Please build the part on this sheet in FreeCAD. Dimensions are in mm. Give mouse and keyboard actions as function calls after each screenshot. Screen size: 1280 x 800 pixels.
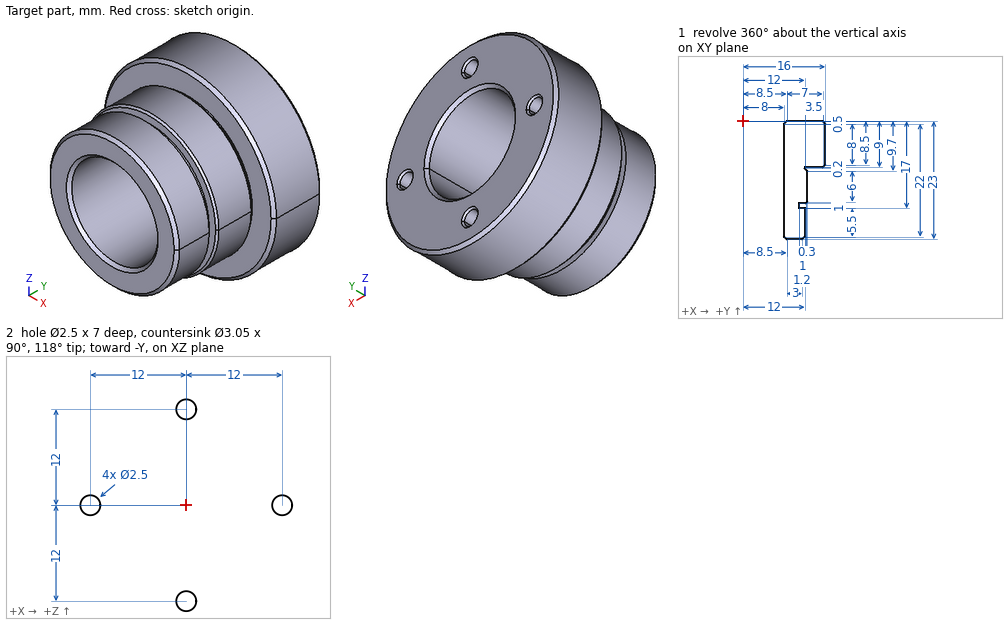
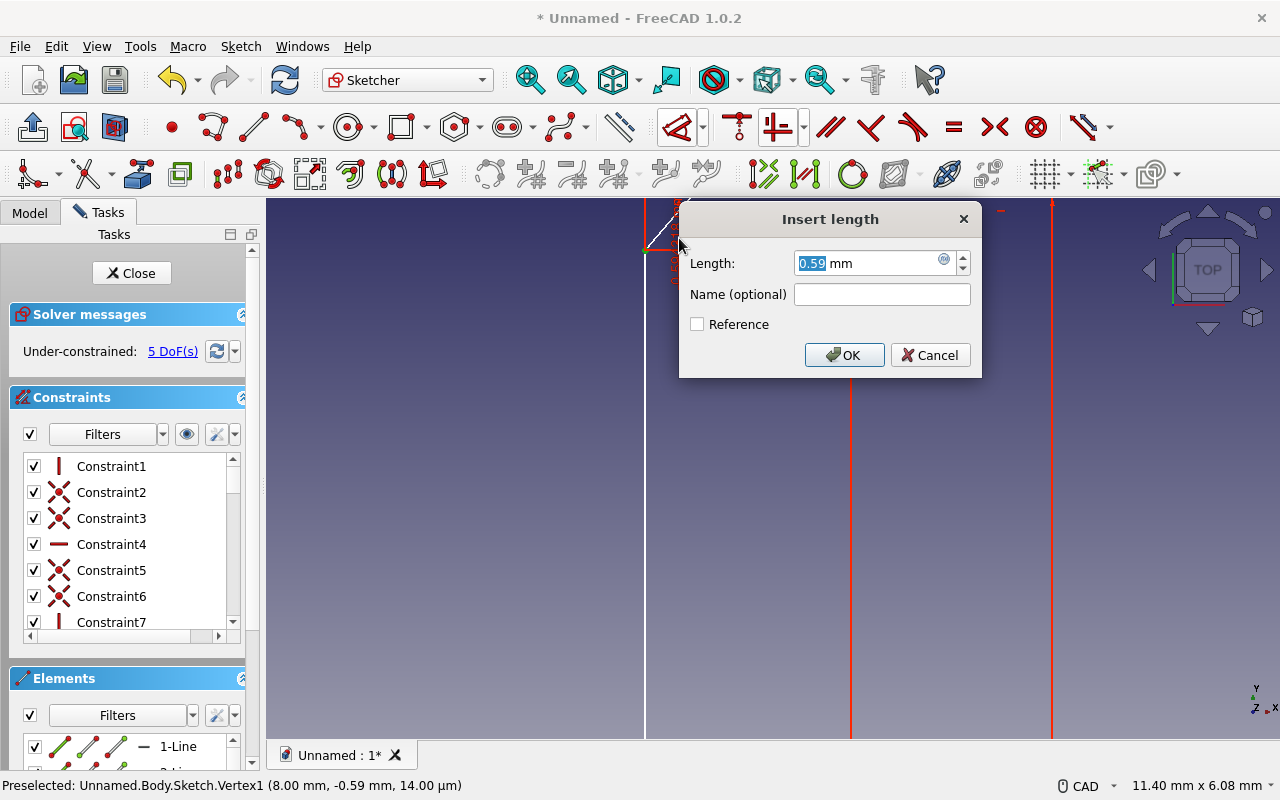
text(0.5)
key(Return)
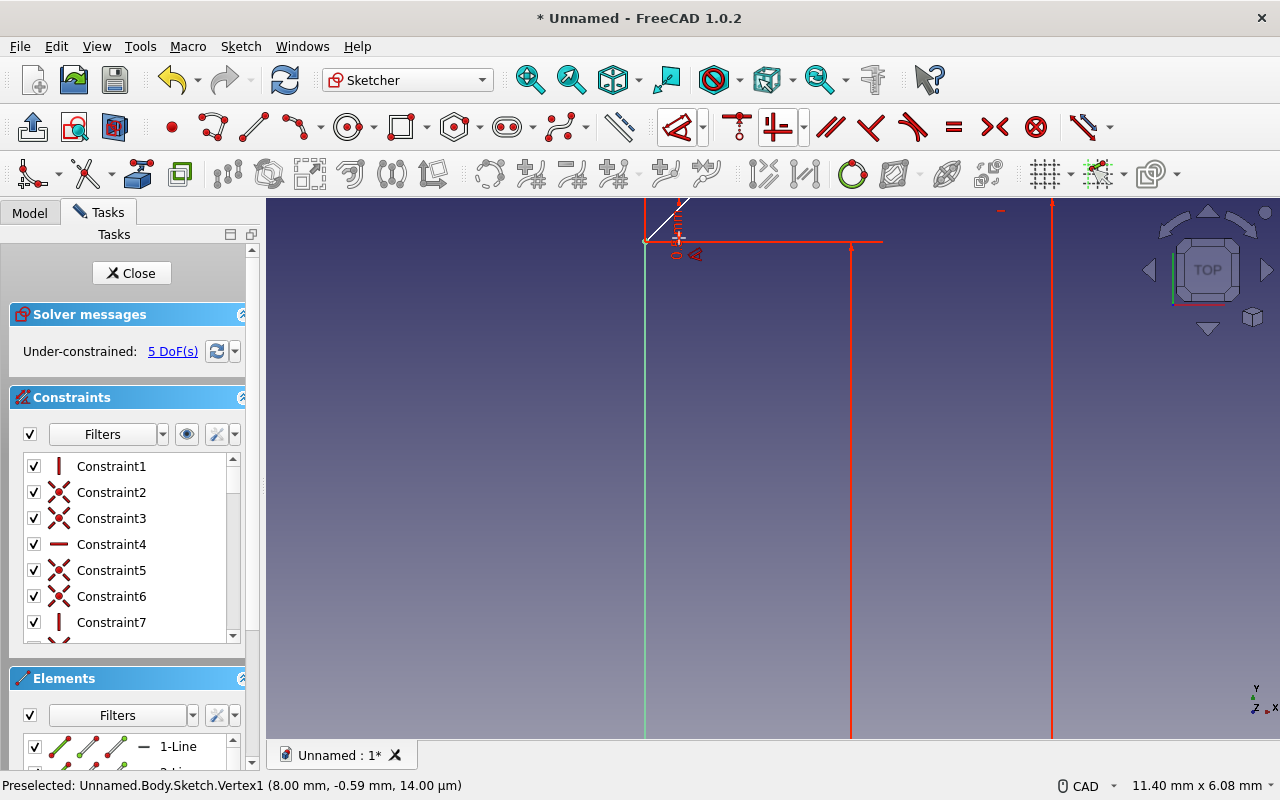
scroll(716, 320, down, 9)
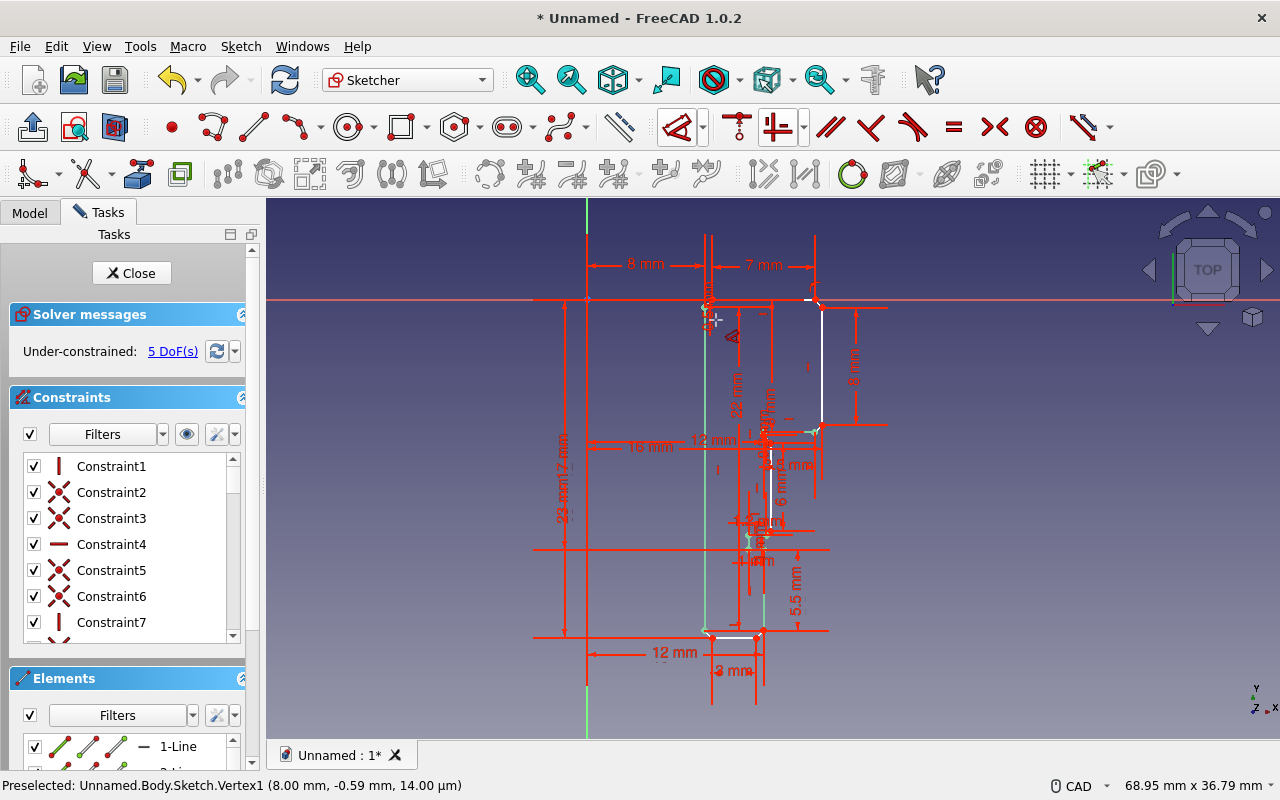
click(712, 638)
click(650, 696)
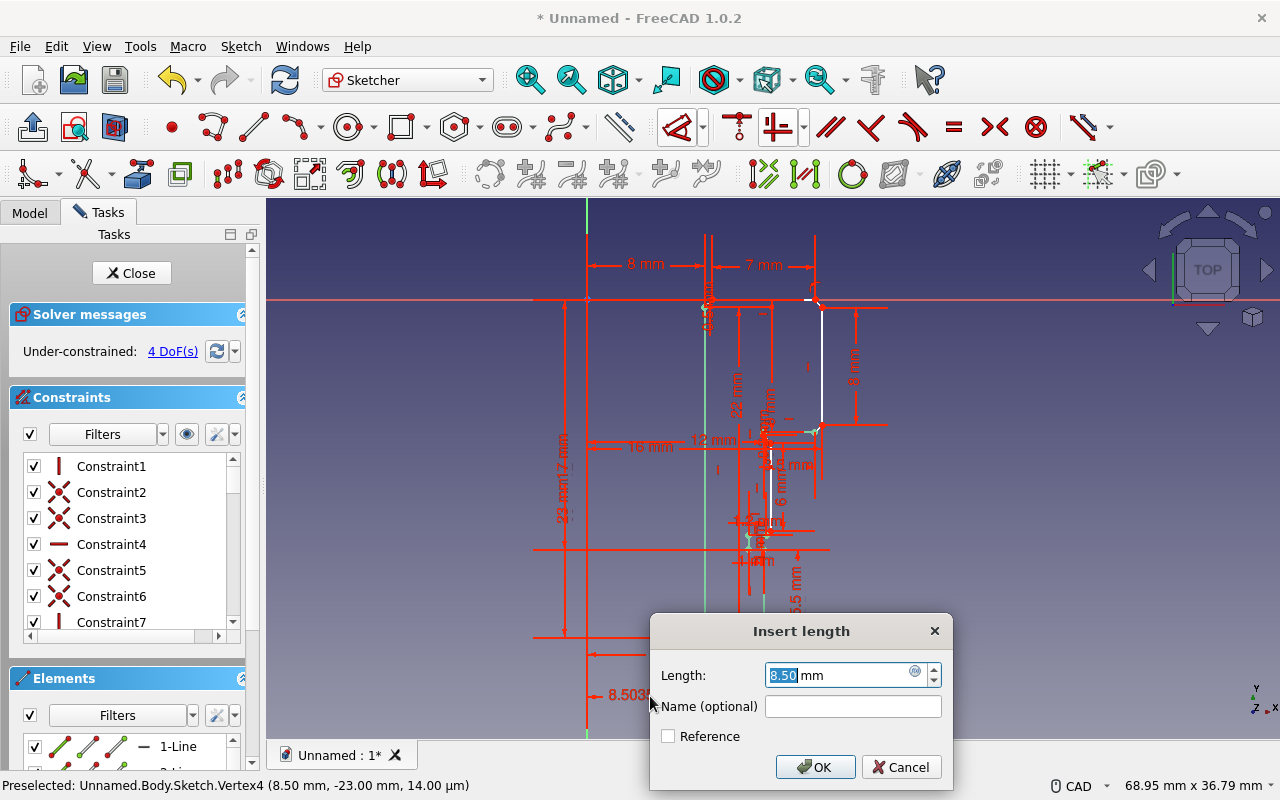
text(8.5)
key(Return)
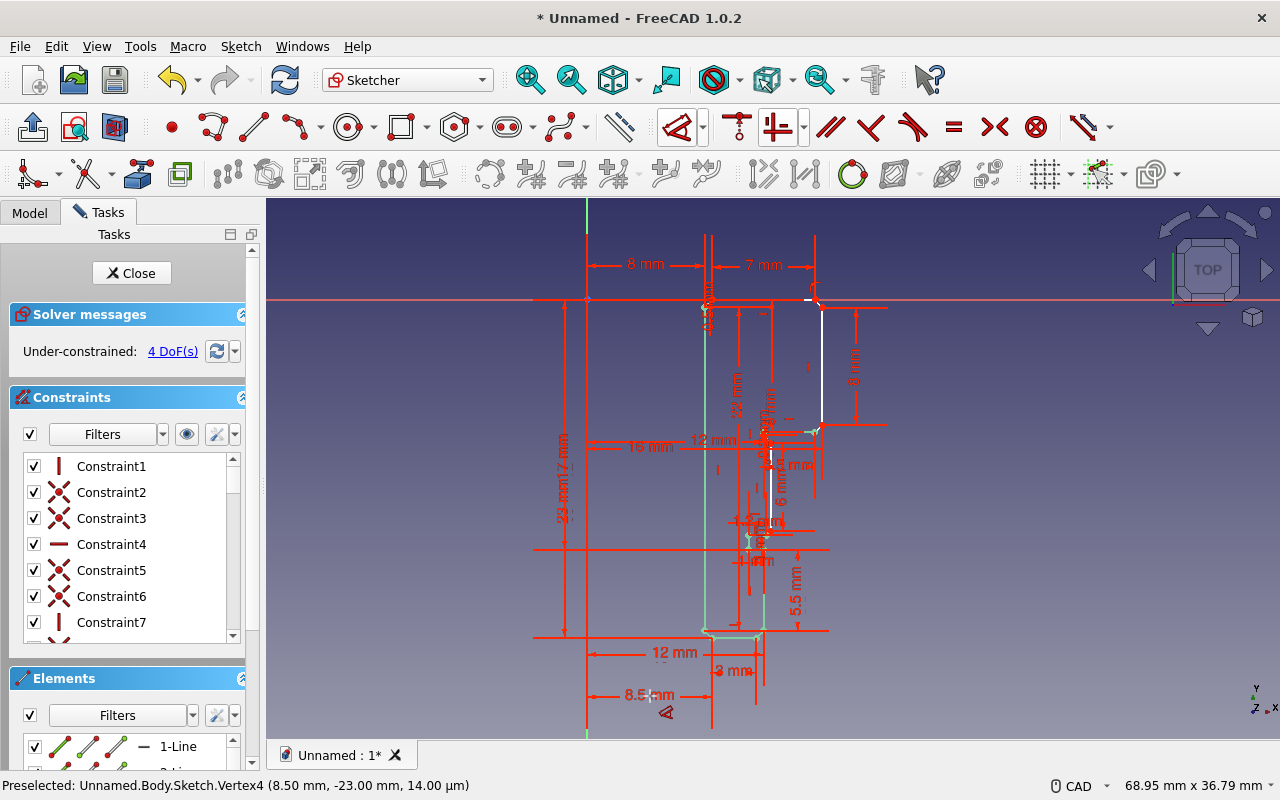
click(771, 443)
click(553, 372)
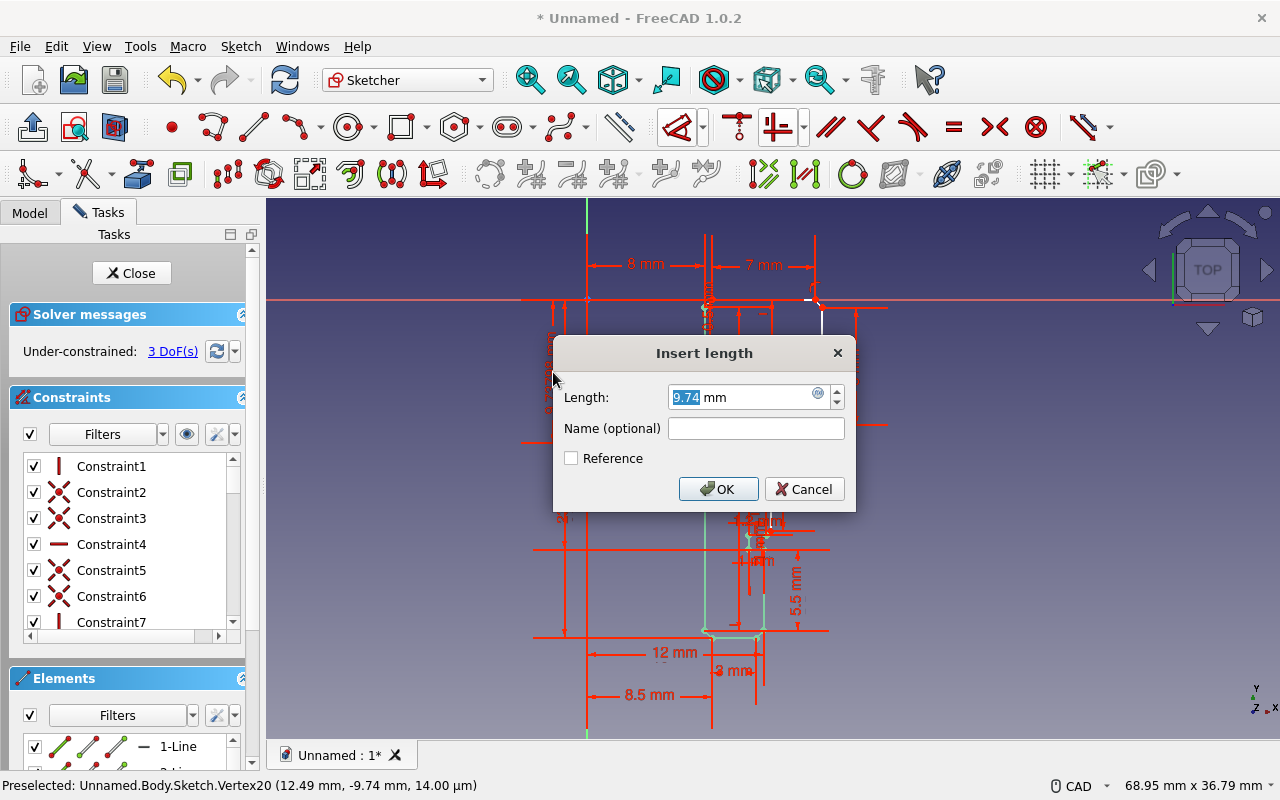
text(9.7)
key(Return)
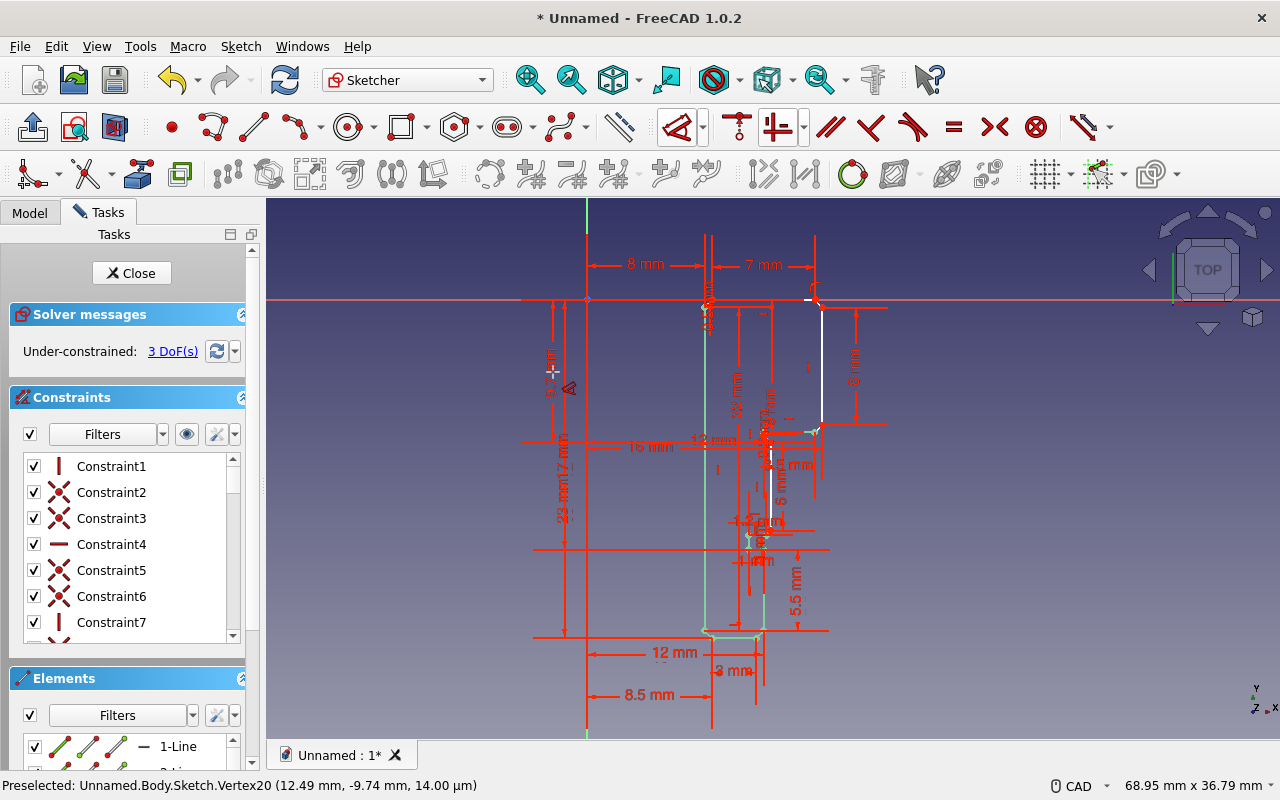
scroll(822, 425, up, 2)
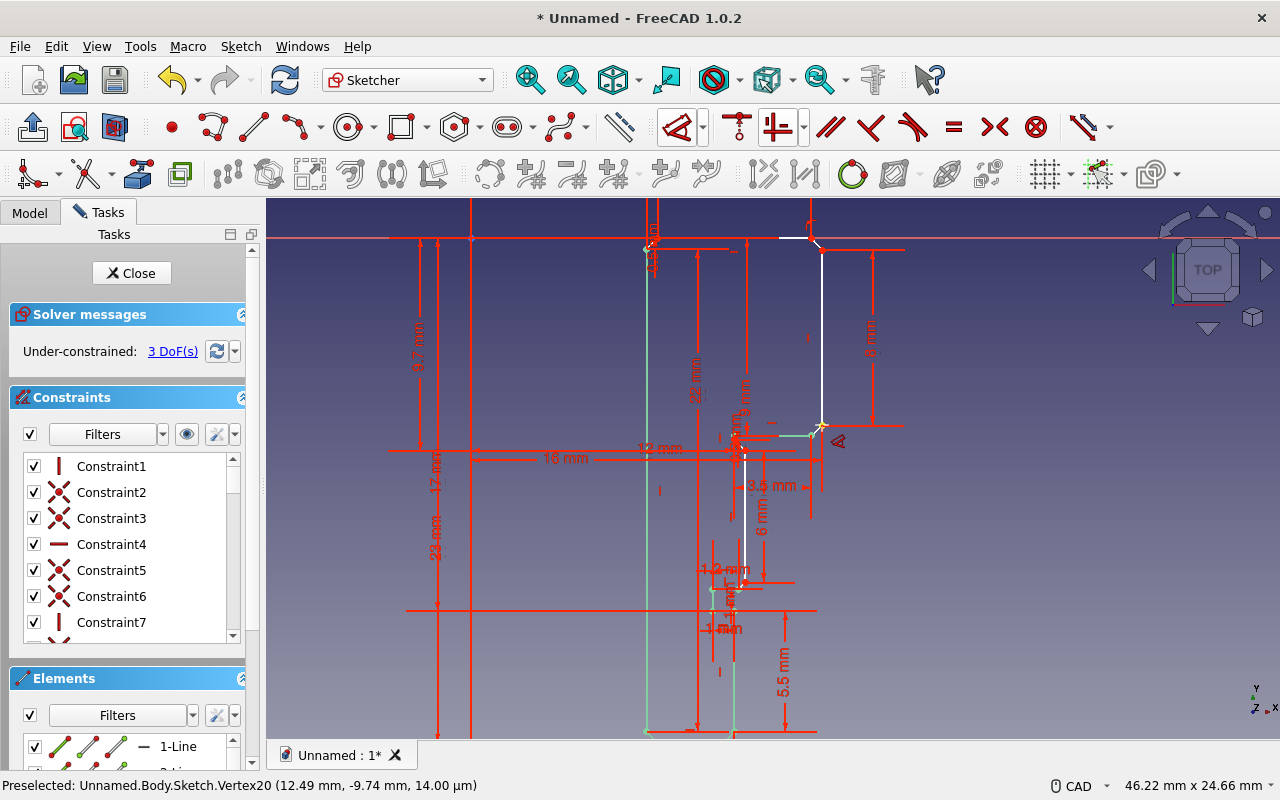
click(822, 426)
click(856, 289)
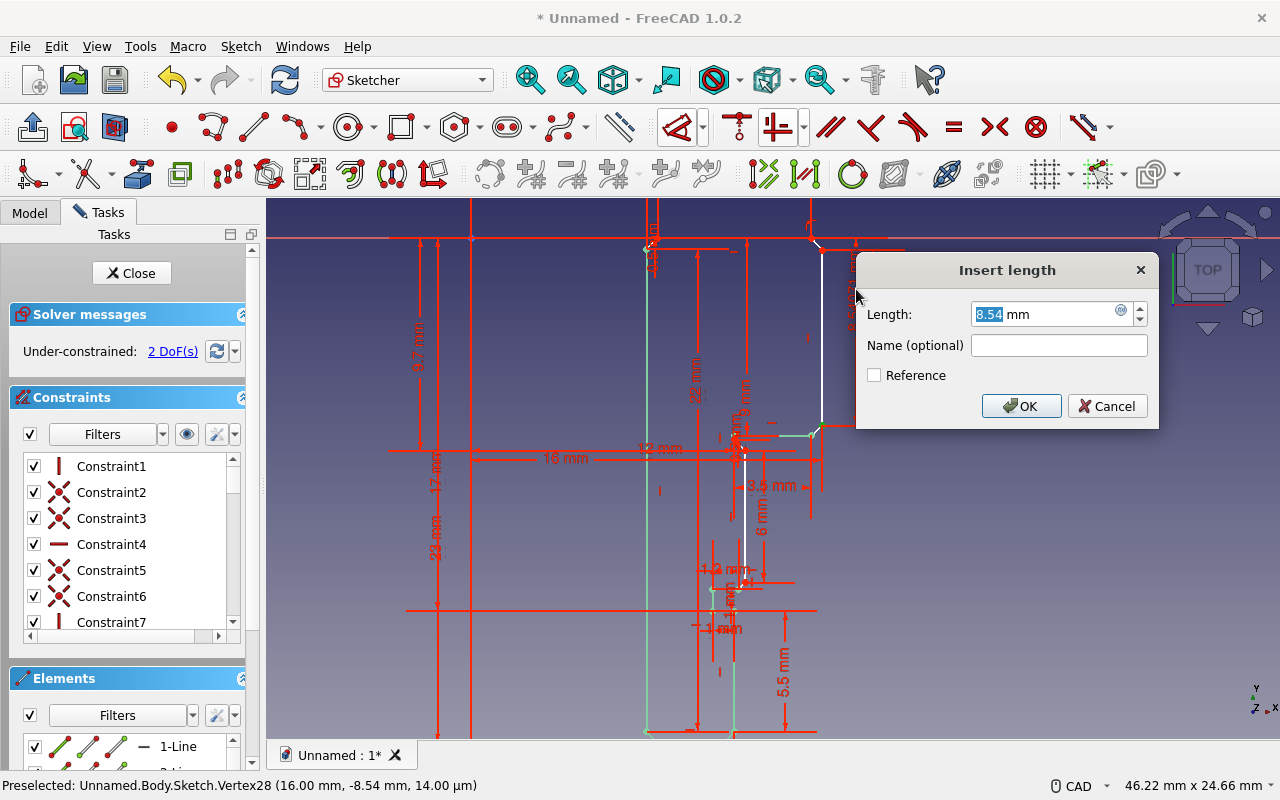
text(8.5)
key(Return)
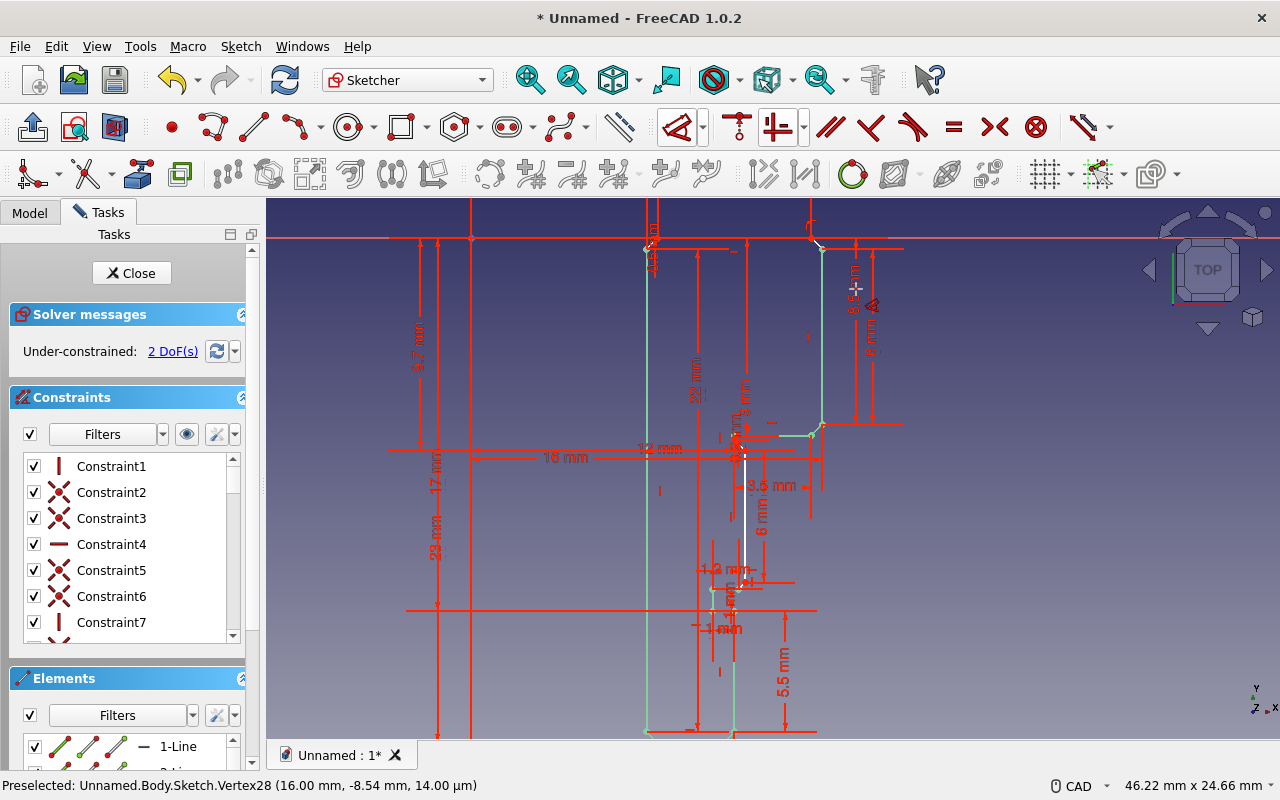
click(658, 238)
click(565, 272)